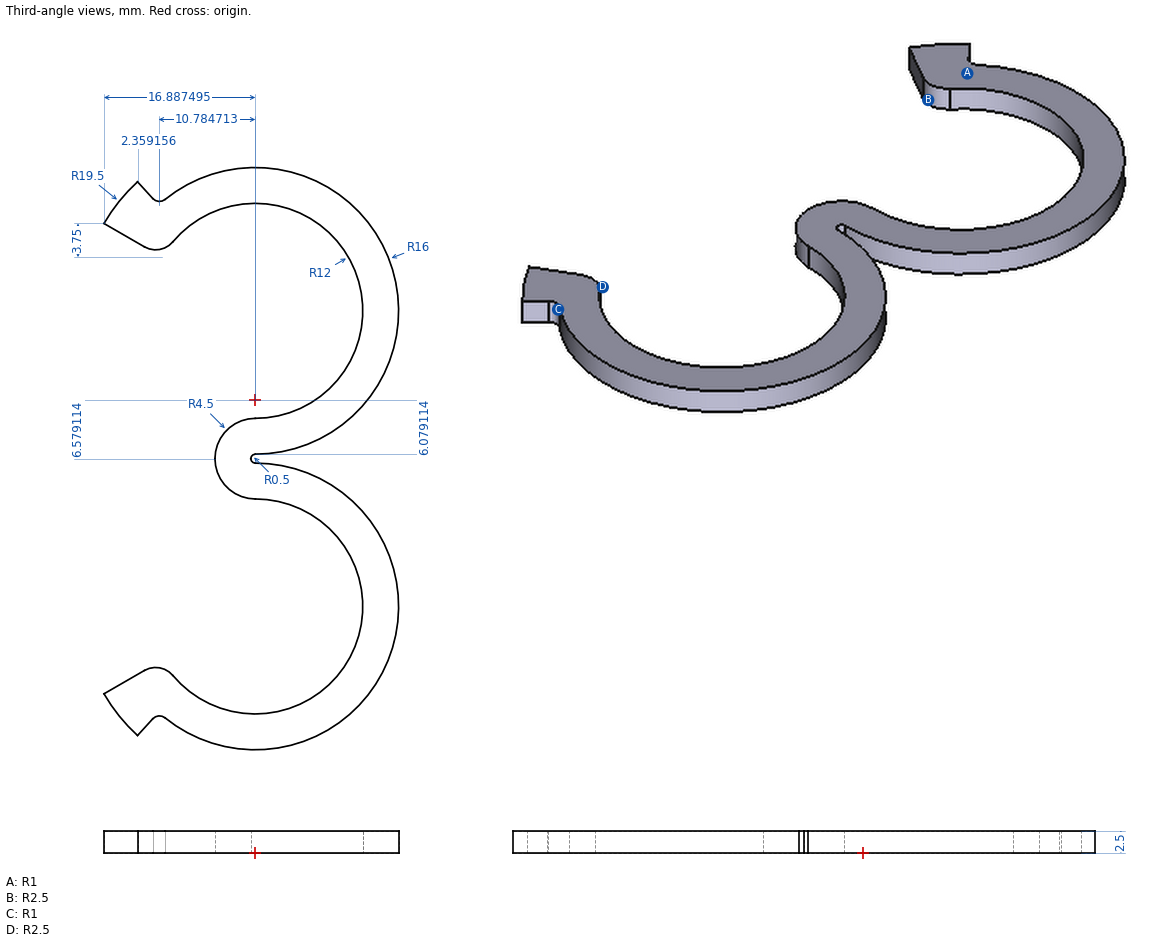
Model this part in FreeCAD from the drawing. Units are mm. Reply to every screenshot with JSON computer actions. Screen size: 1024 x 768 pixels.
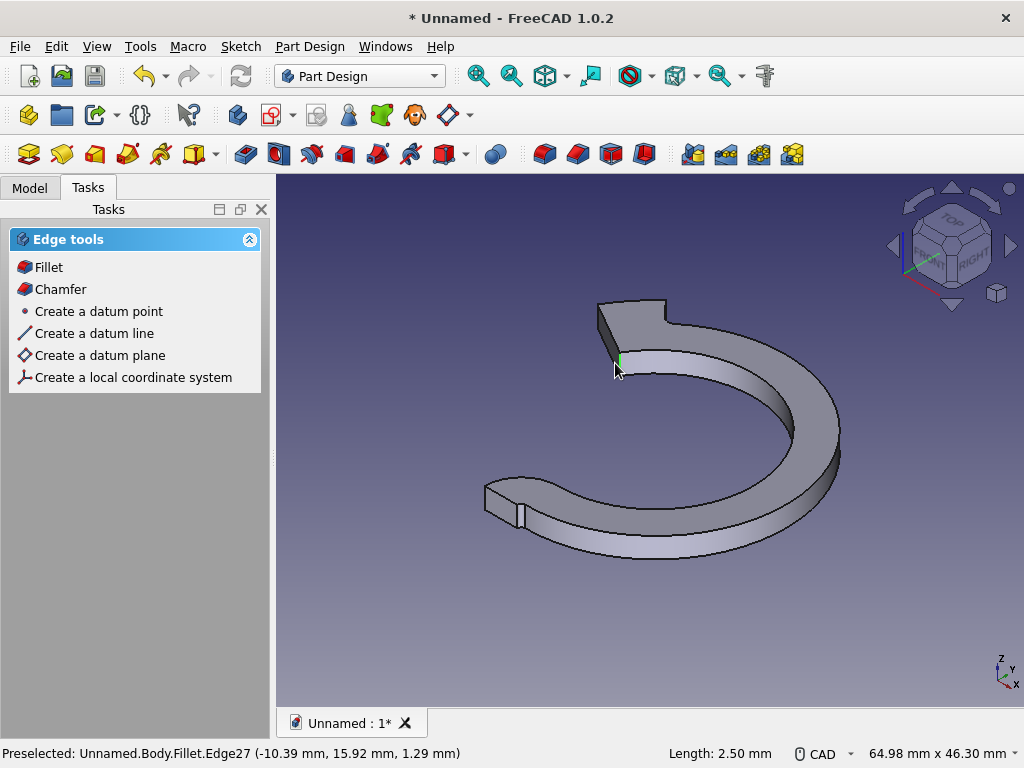
{"action": "left_click", "coordinate": [545, 154]}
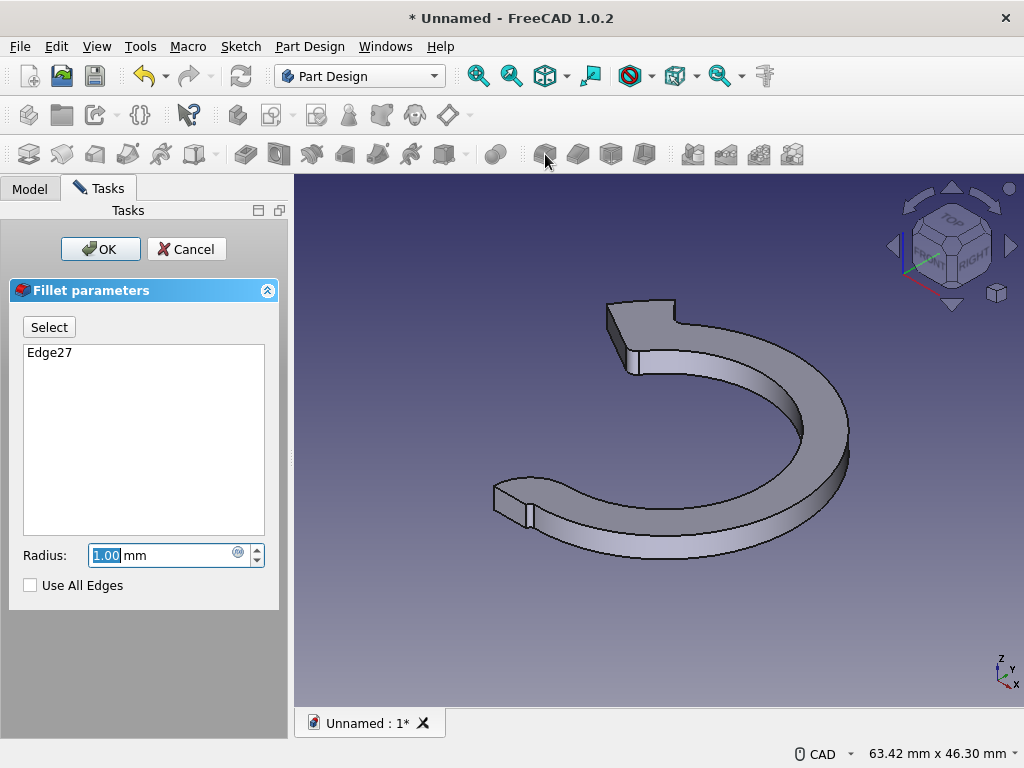
{"action": "type", "text": "2.5"}
{"action": "key", "text": "Tab"}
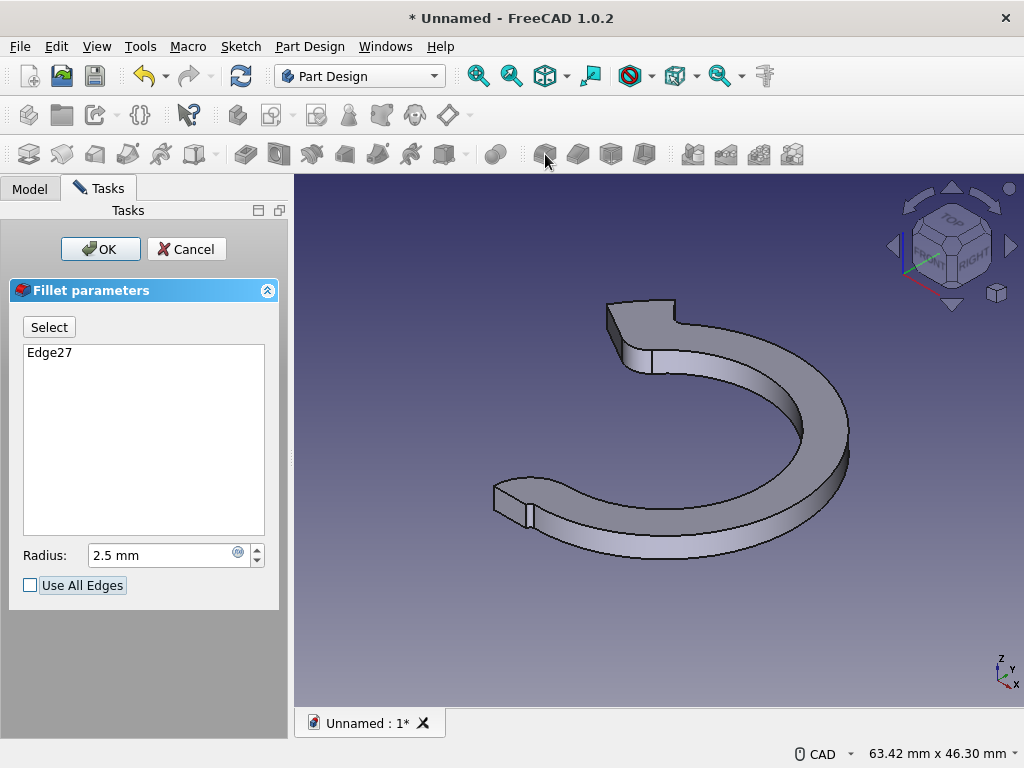
{"action": "left_click", "coordinate": [101, 249]}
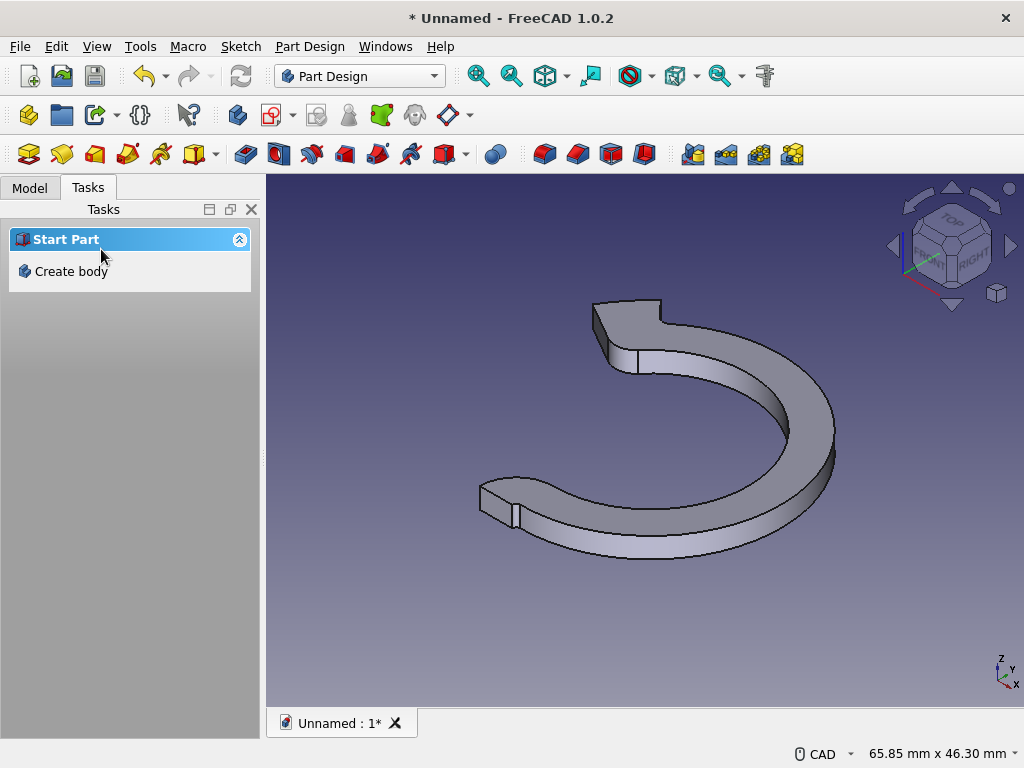
{"action": "left_click", "coordinate": [30, 188]}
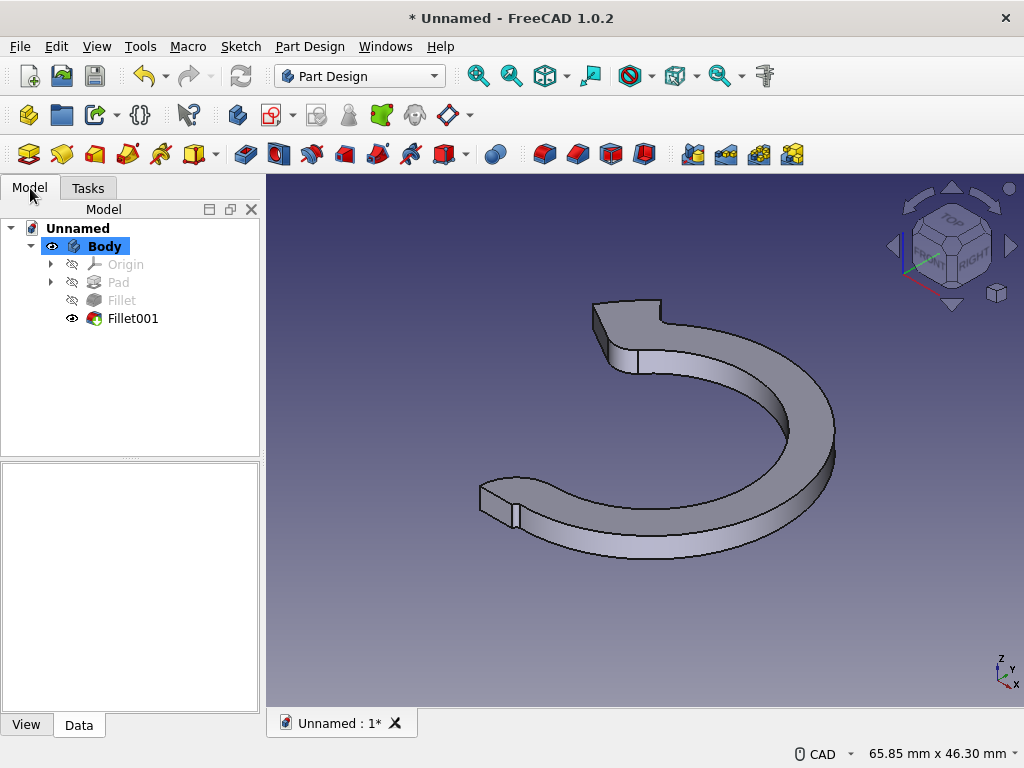
{"action": "left_click", "coordinate": [51, 264]}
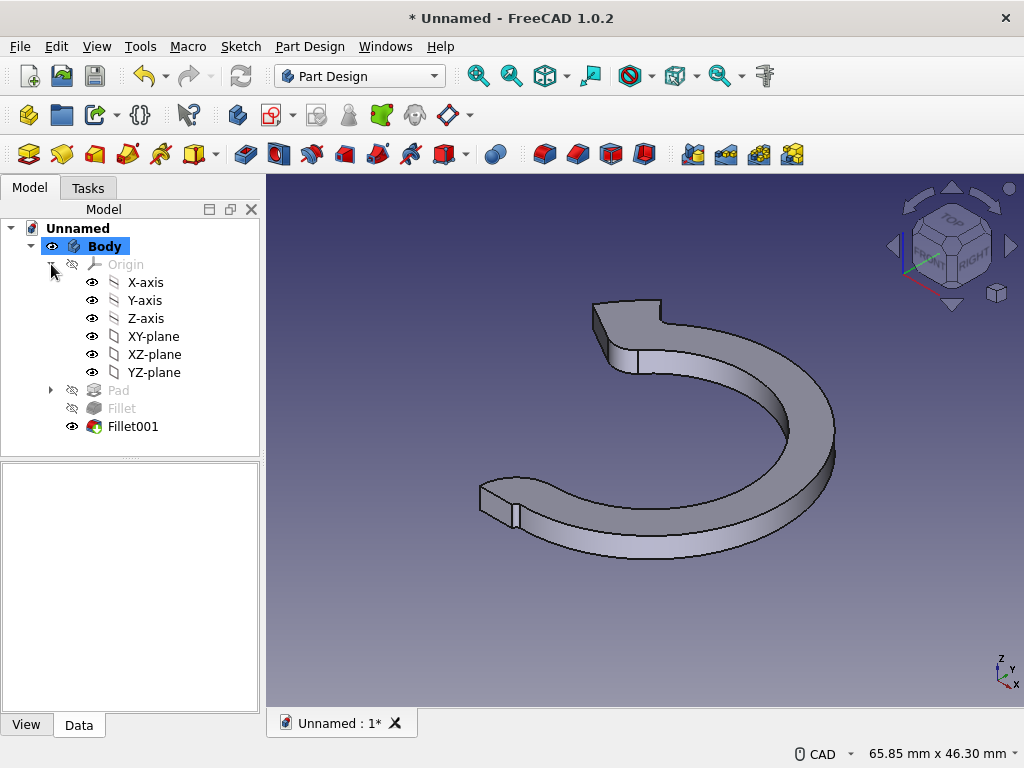
{"action": "left_click", "coordinate": [137, 354]}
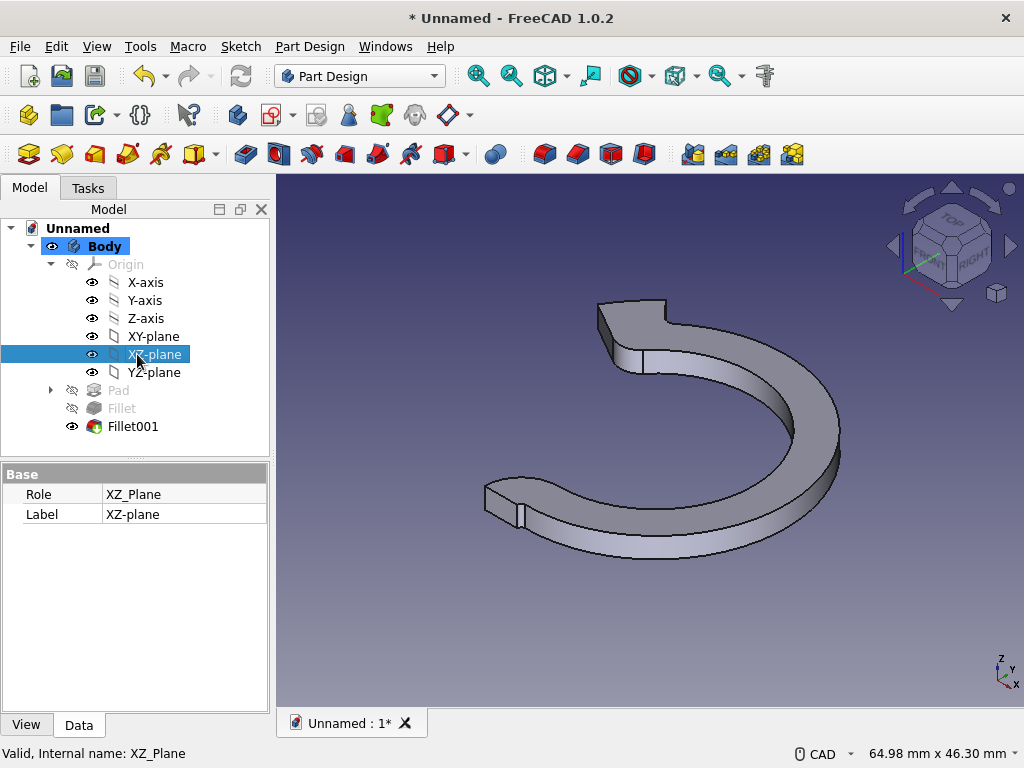
{"action": "left_click", "coordinate": [448, 116]}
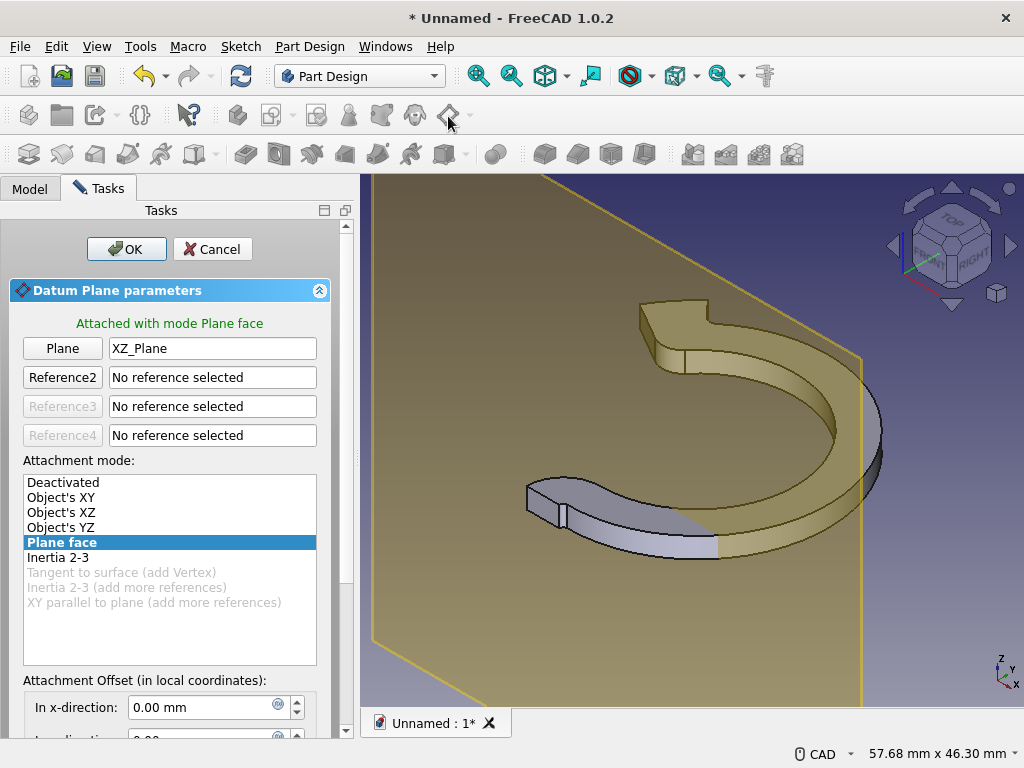
{"action": "scroll", "coordinate": [346, 479], "scroll_direction": "down", "scroll_amount": 2}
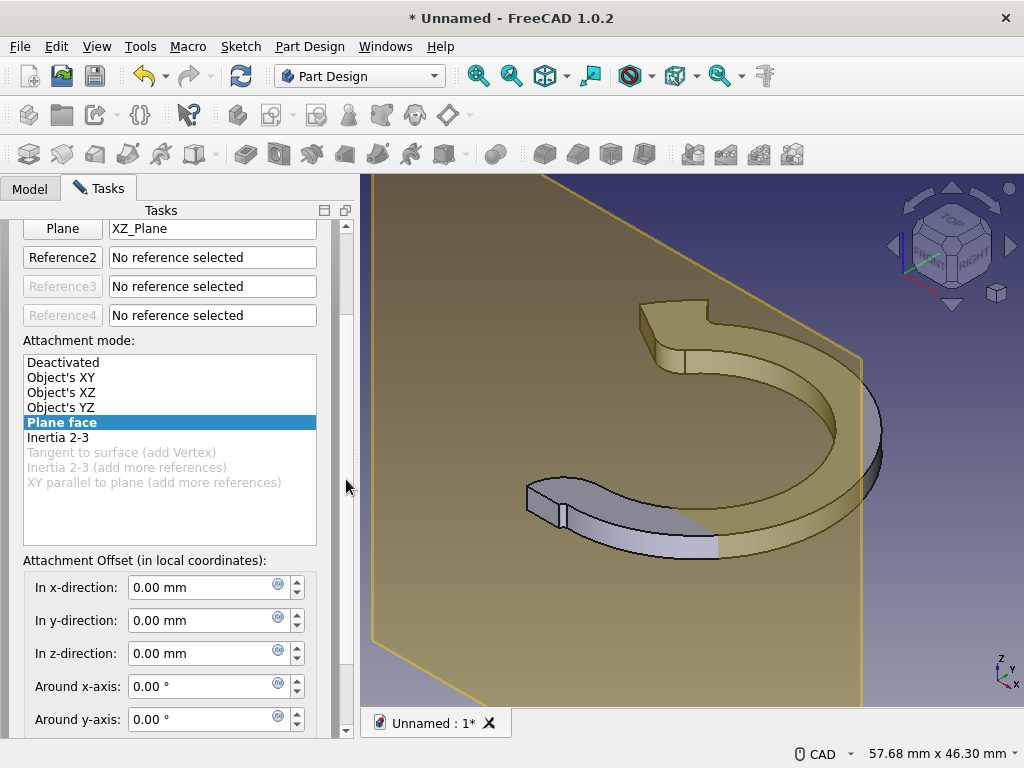
{"action": "triple_click", "coordinate": [210, 654]}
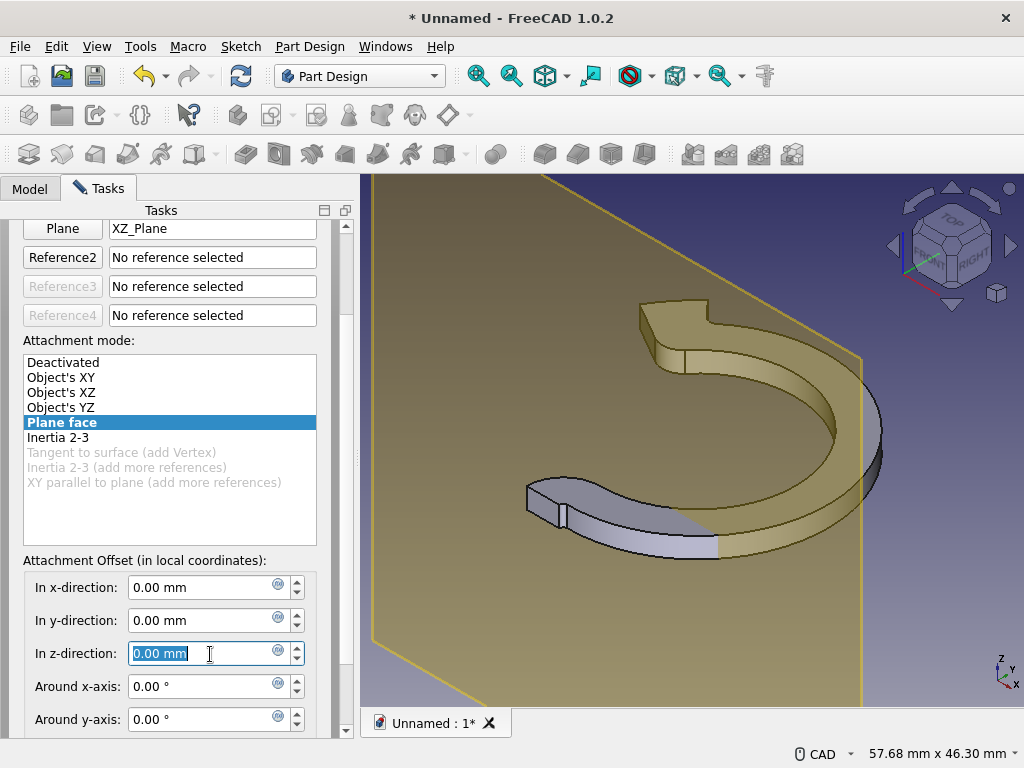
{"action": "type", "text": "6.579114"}
{"action": "key", "text": "Tab"}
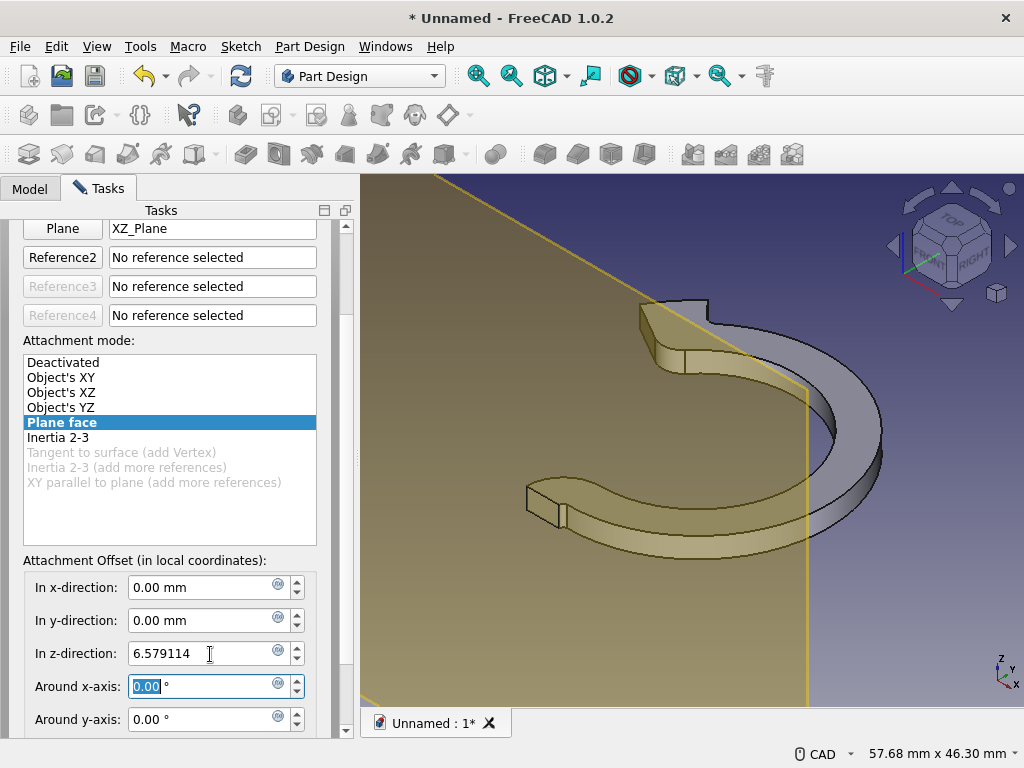
{"action": "scroll", "coordinate": [346, 479], "scroll_direction": "up", "scroll_amount": 3}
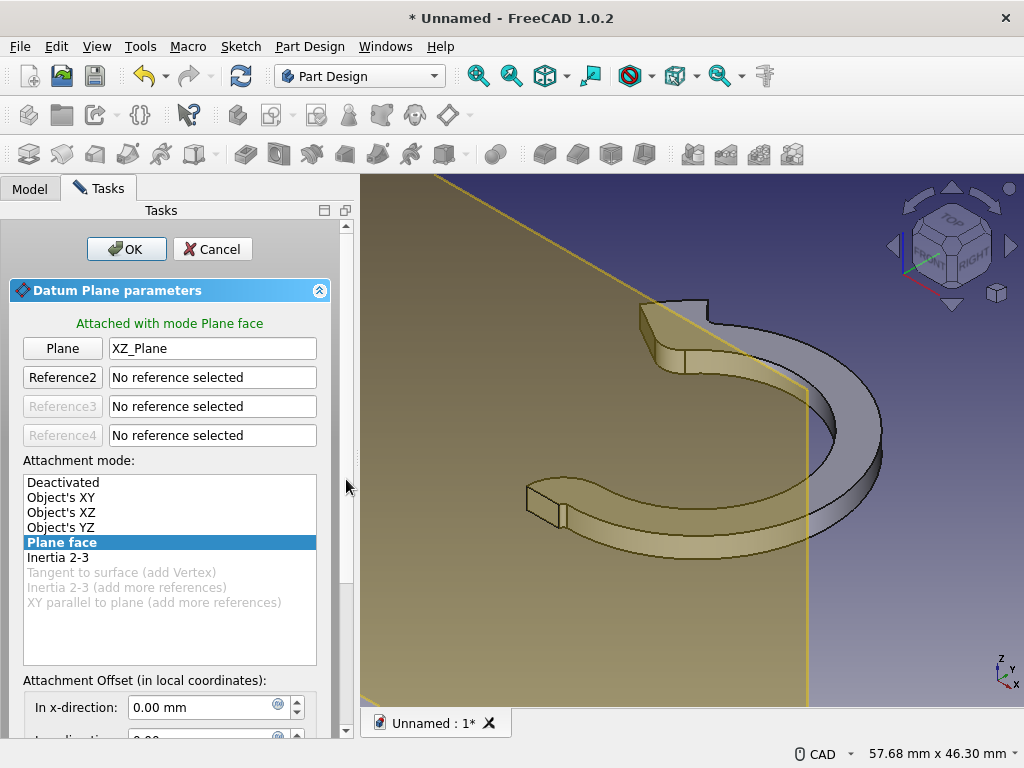
{"action": "left_click", "coordinate": [127, 249]}